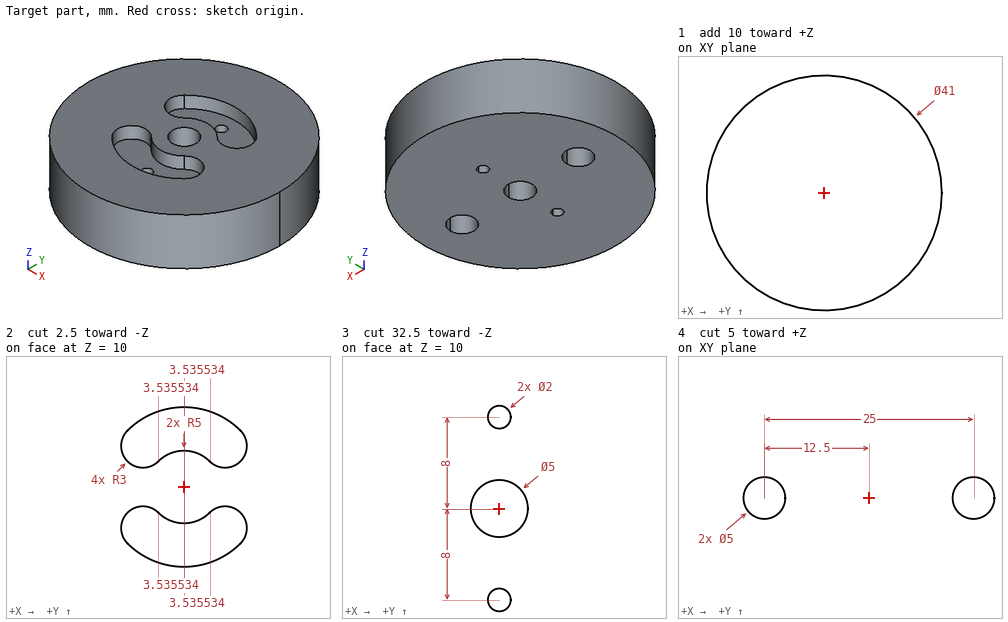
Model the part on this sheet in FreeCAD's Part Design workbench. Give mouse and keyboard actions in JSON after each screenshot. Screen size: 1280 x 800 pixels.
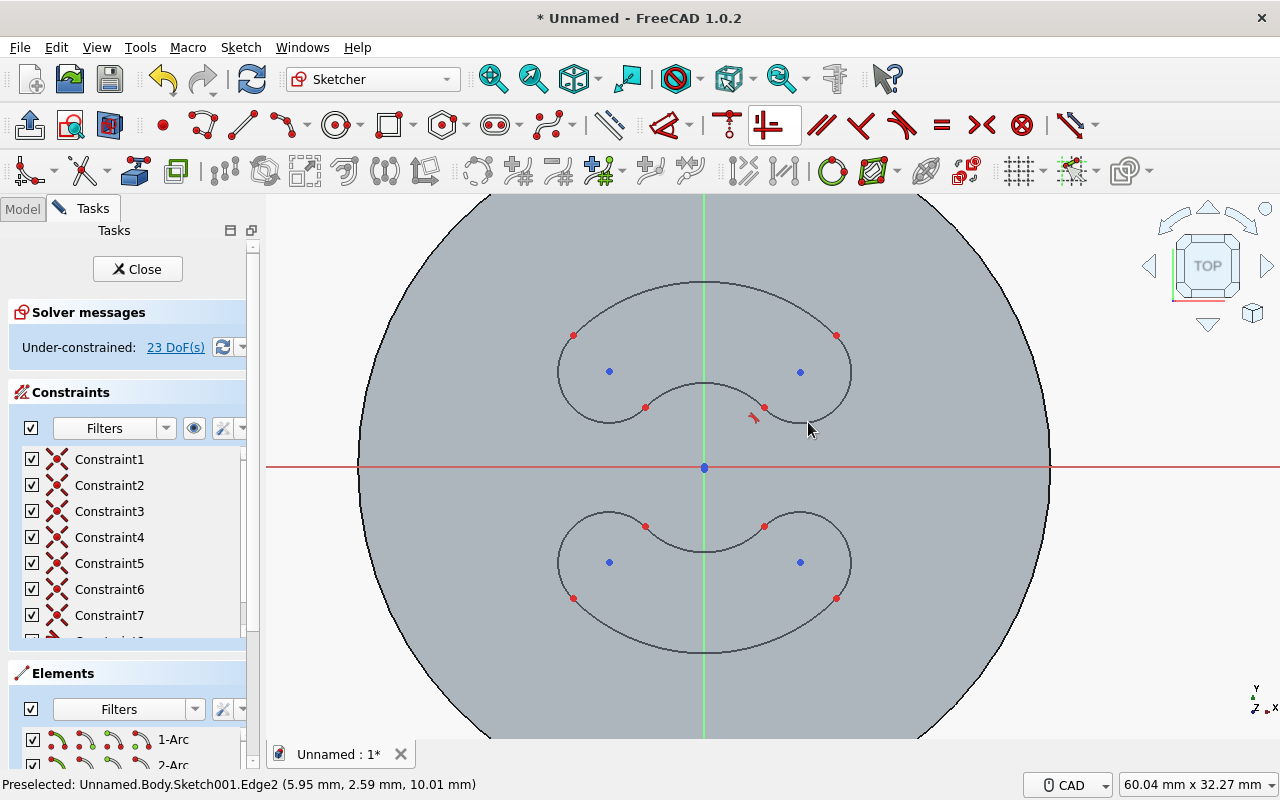
{"action": "left_click", "coordinate": [731, 387]}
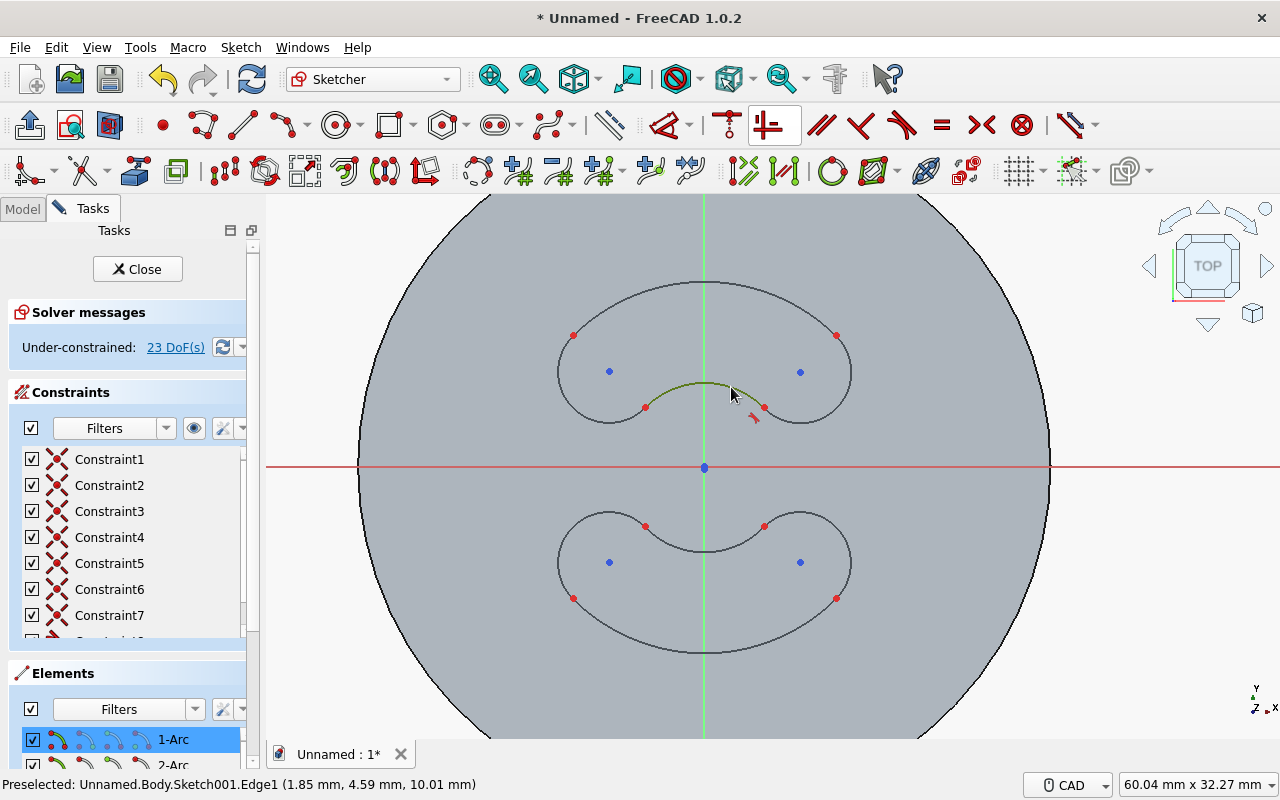
{"action": "left_click", "coordinate": [559, 380]}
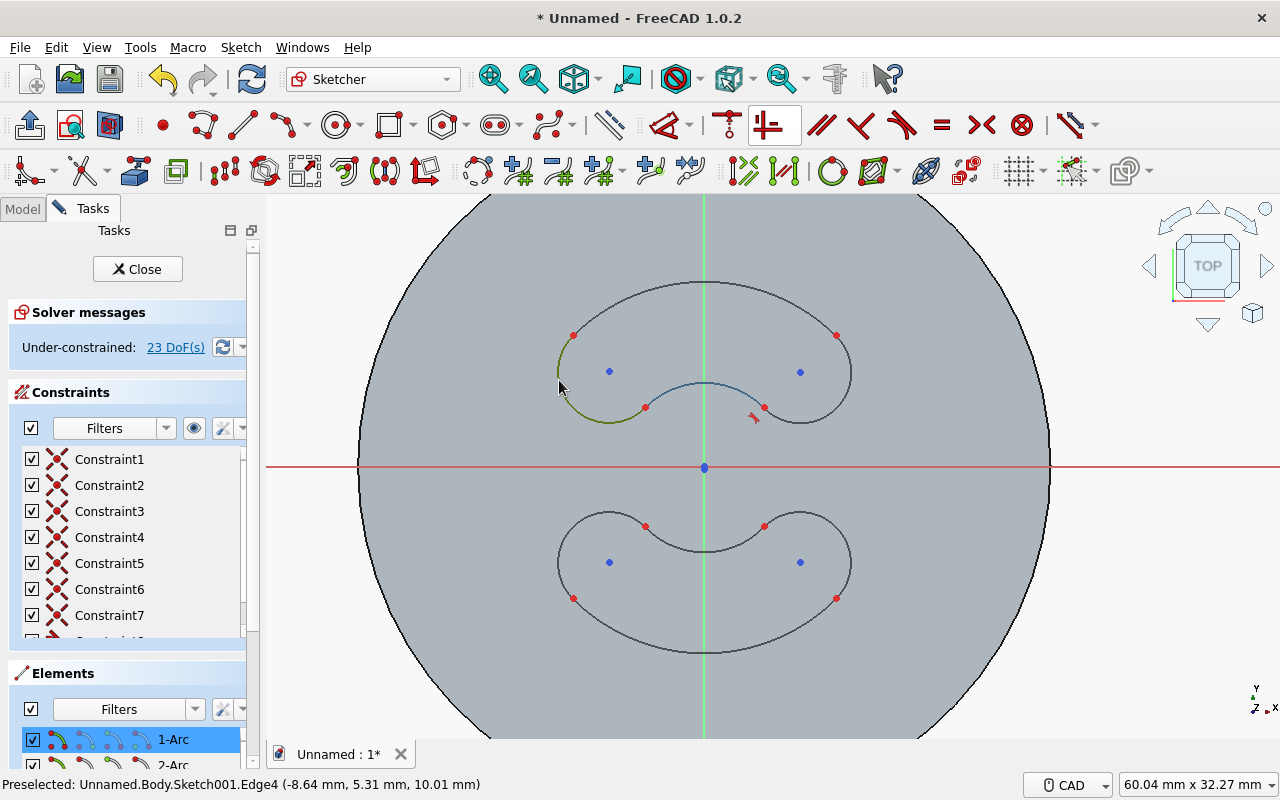
{"action": "key", "text": "t"}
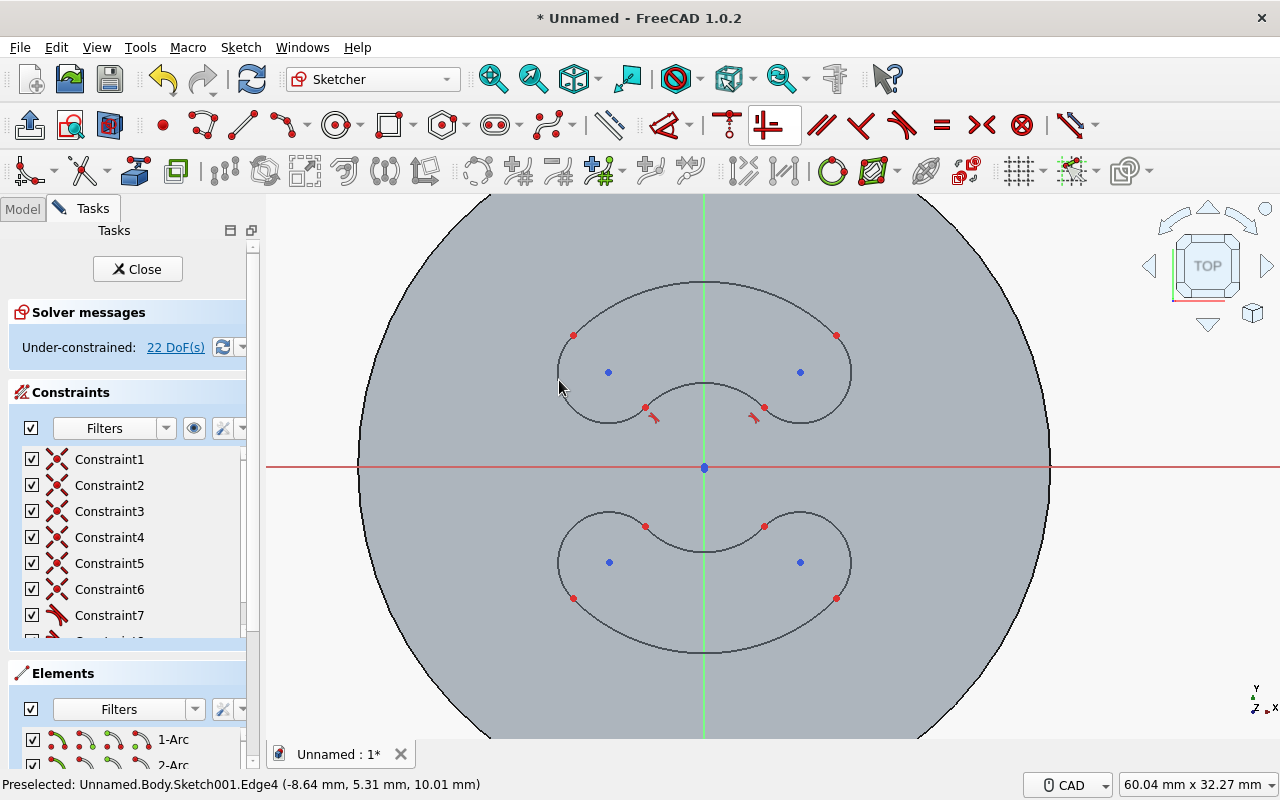
{"action": "left_click", "coordinate": [808, 423]}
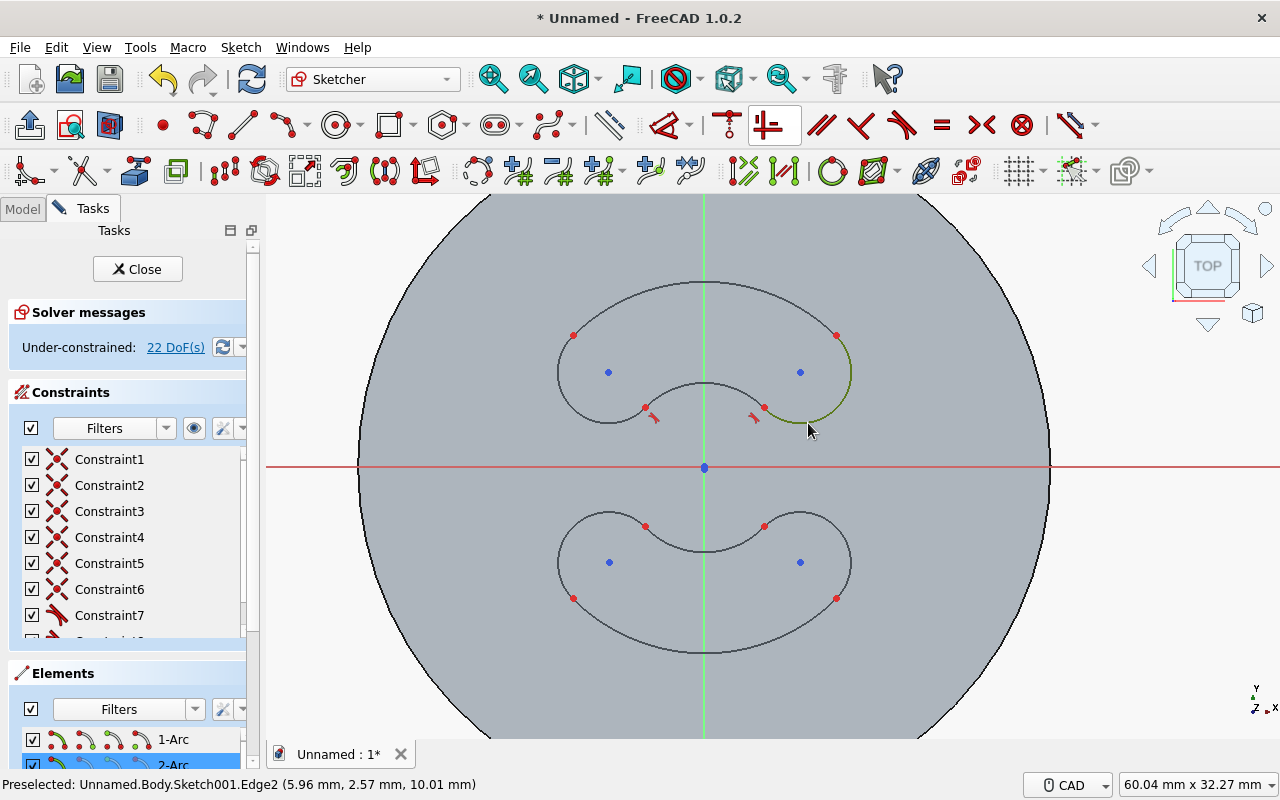
{"action": "left_click", "coordinate": [762, 291]}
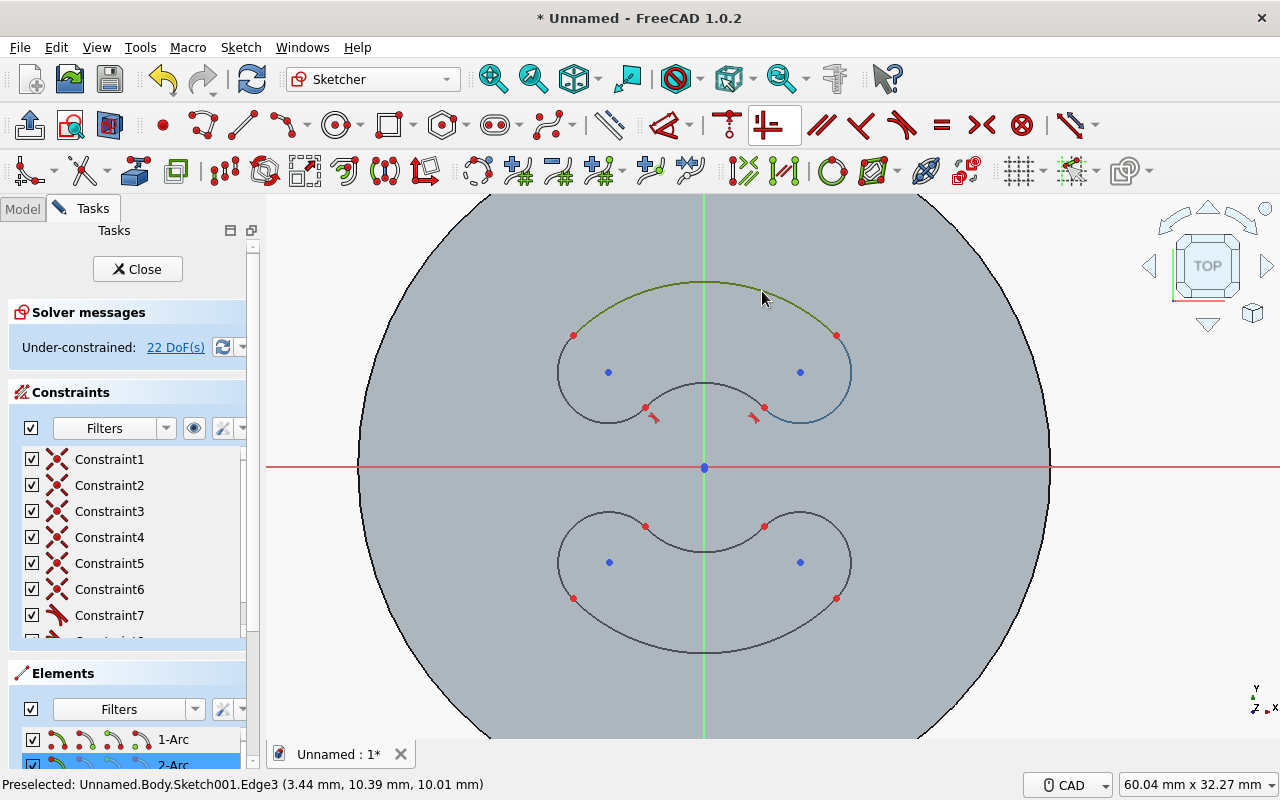
{"action": "left_click", "coordinate": [902, 126]}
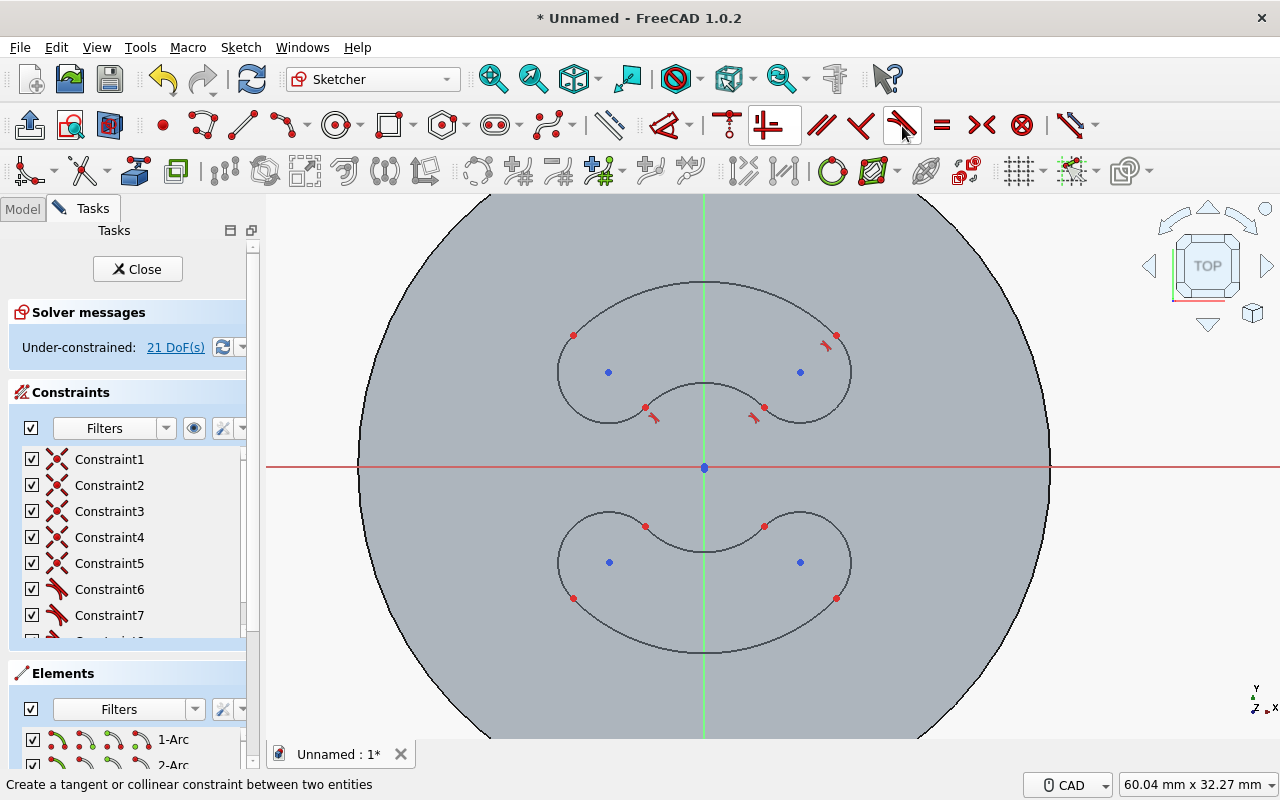
{"action": "left_click", "coordinate": [762, 291]}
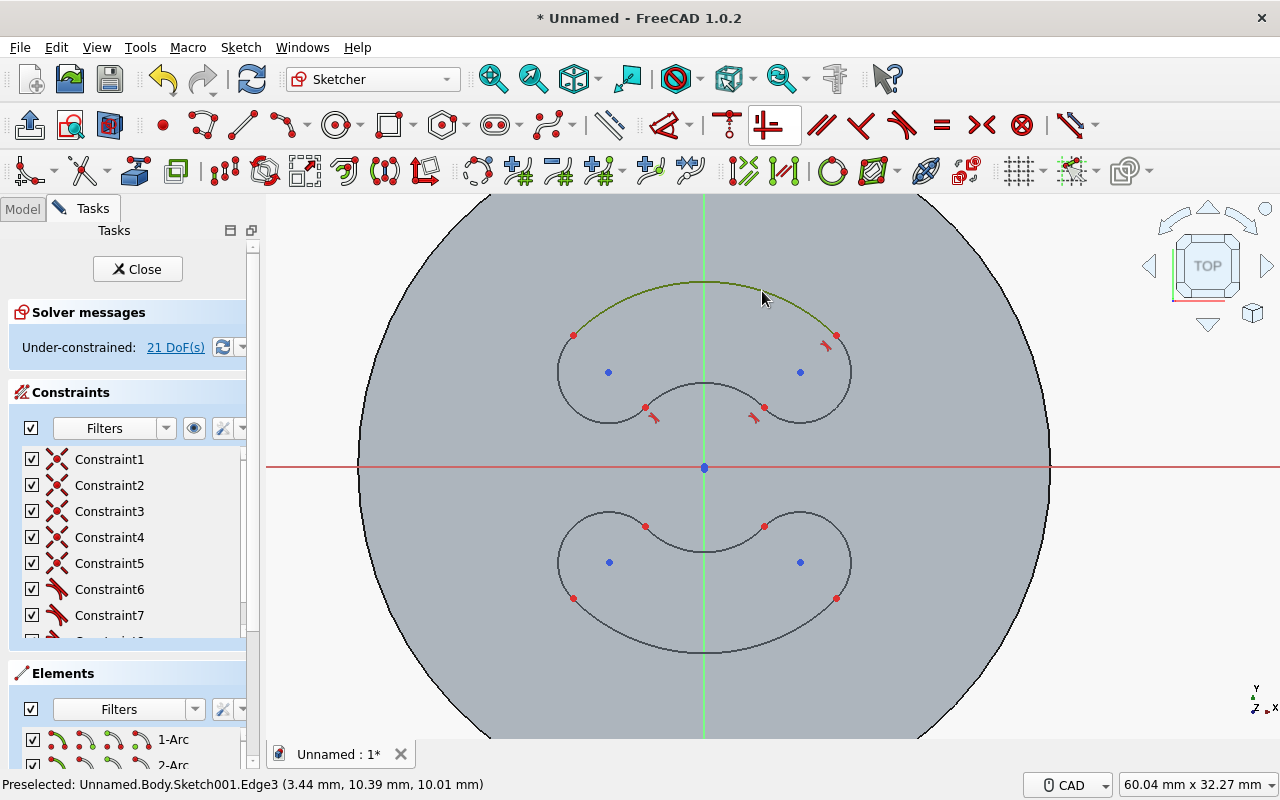
{"action": "left_click", "coordinate": [558, 380]}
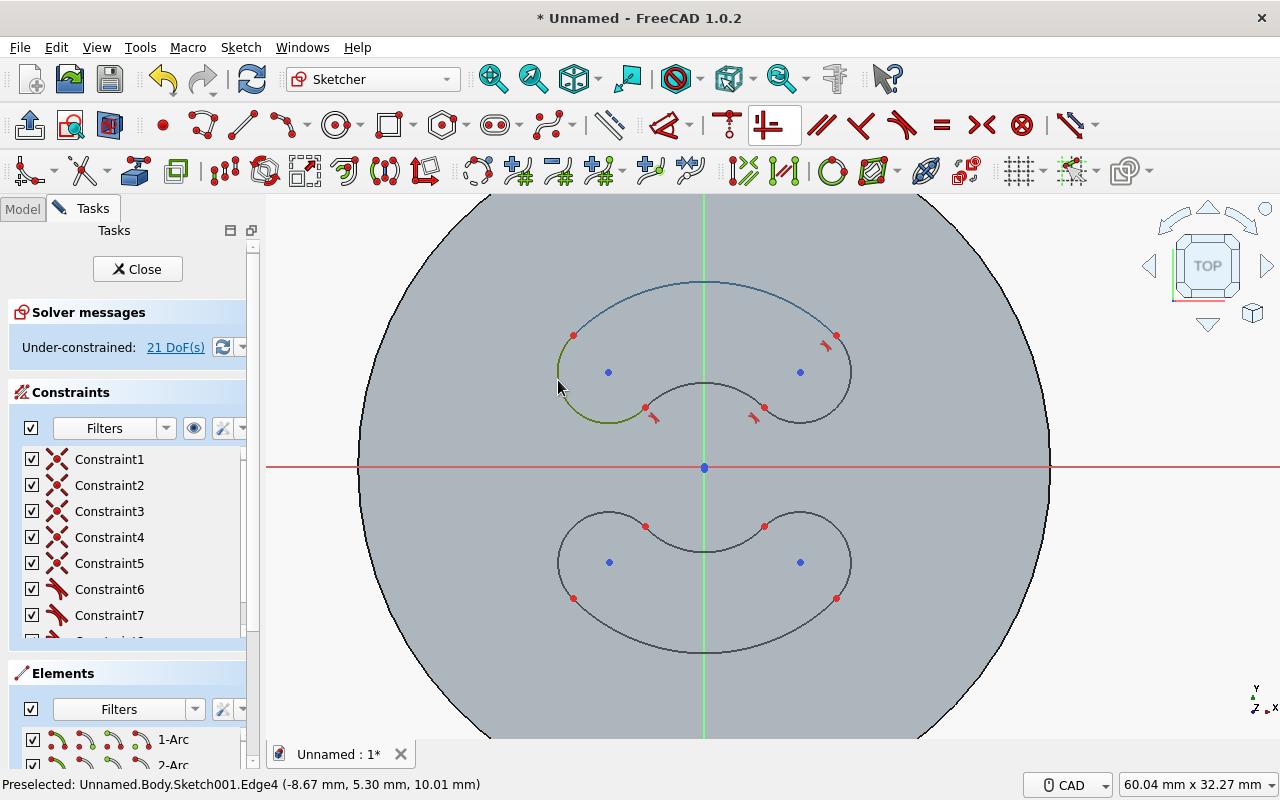
{"action": "key", "text": "t"}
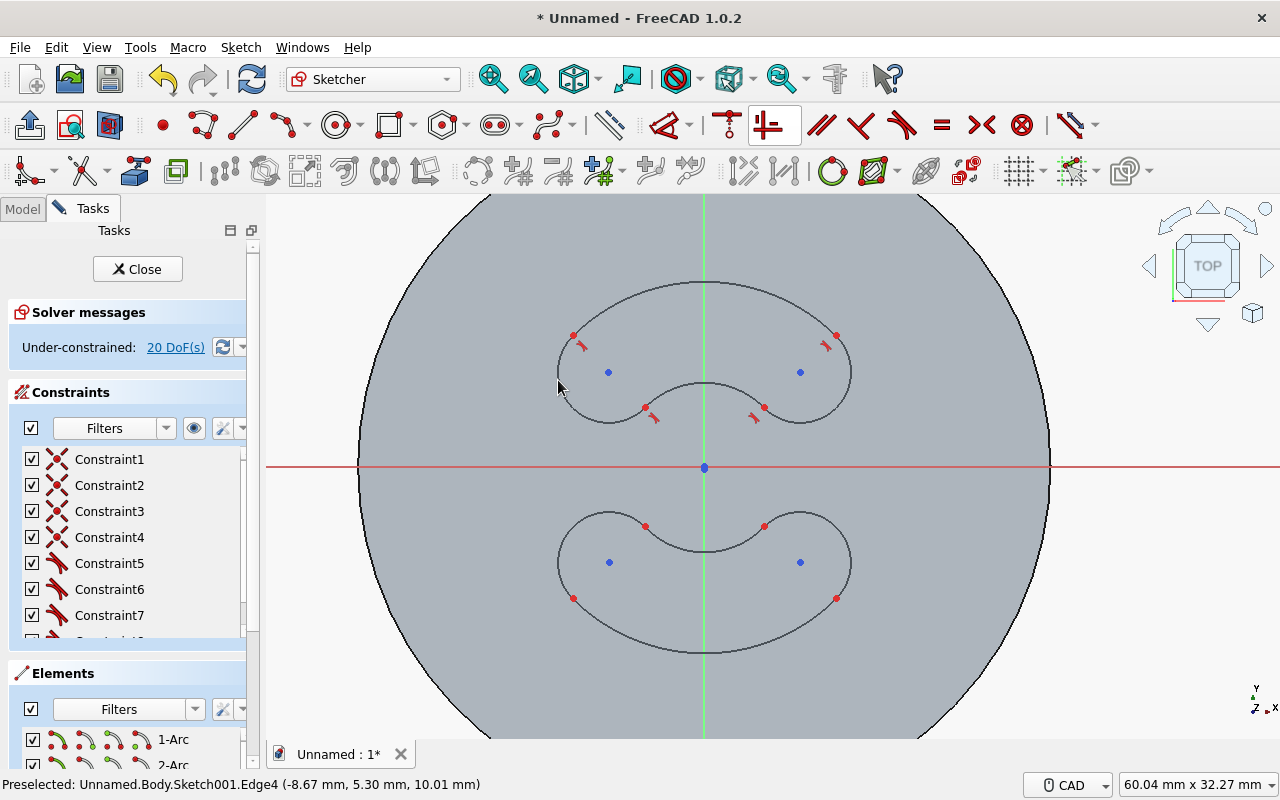
{"action": "left_click", "coordinate": [678, 548]}